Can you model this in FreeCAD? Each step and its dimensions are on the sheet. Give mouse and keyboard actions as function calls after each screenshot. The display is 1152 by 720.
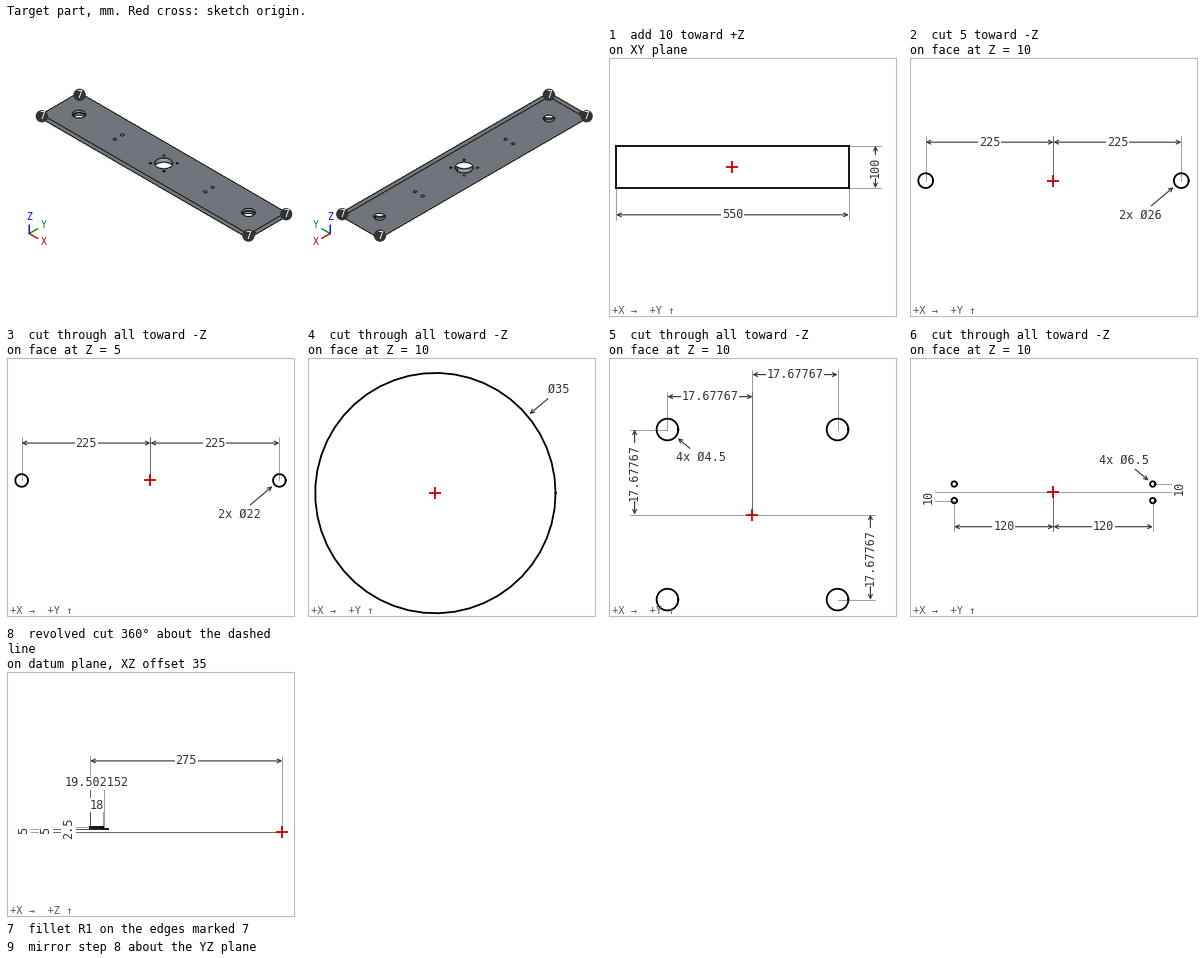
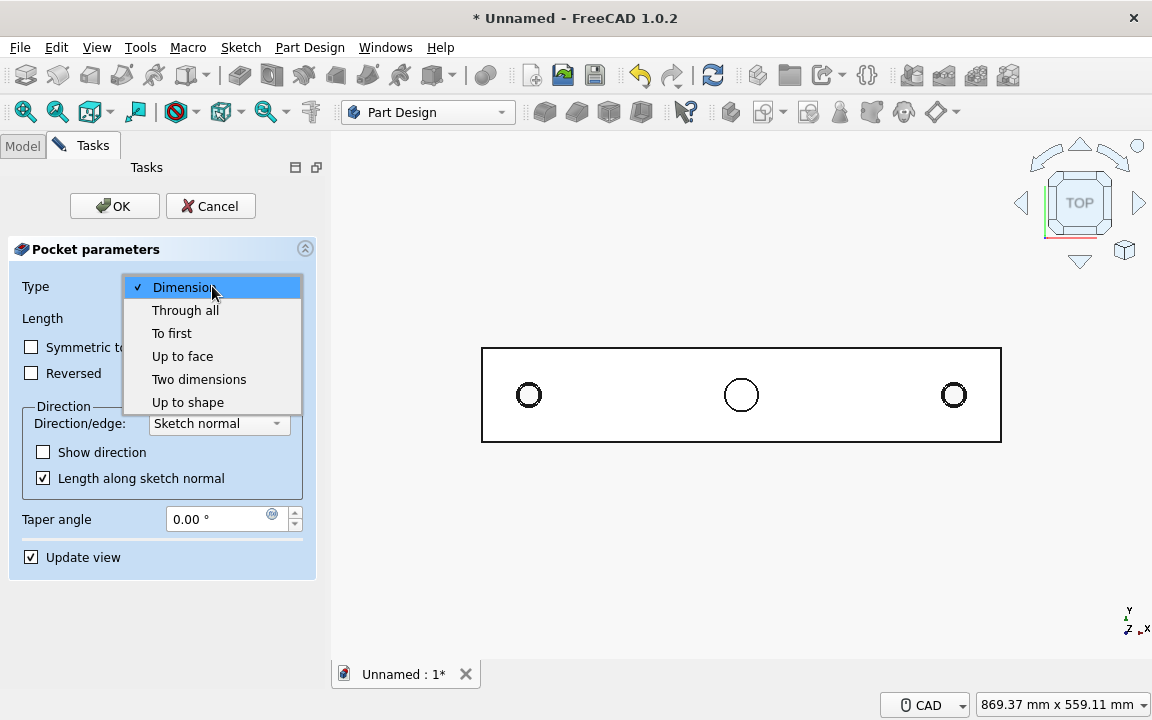
click(212, 310)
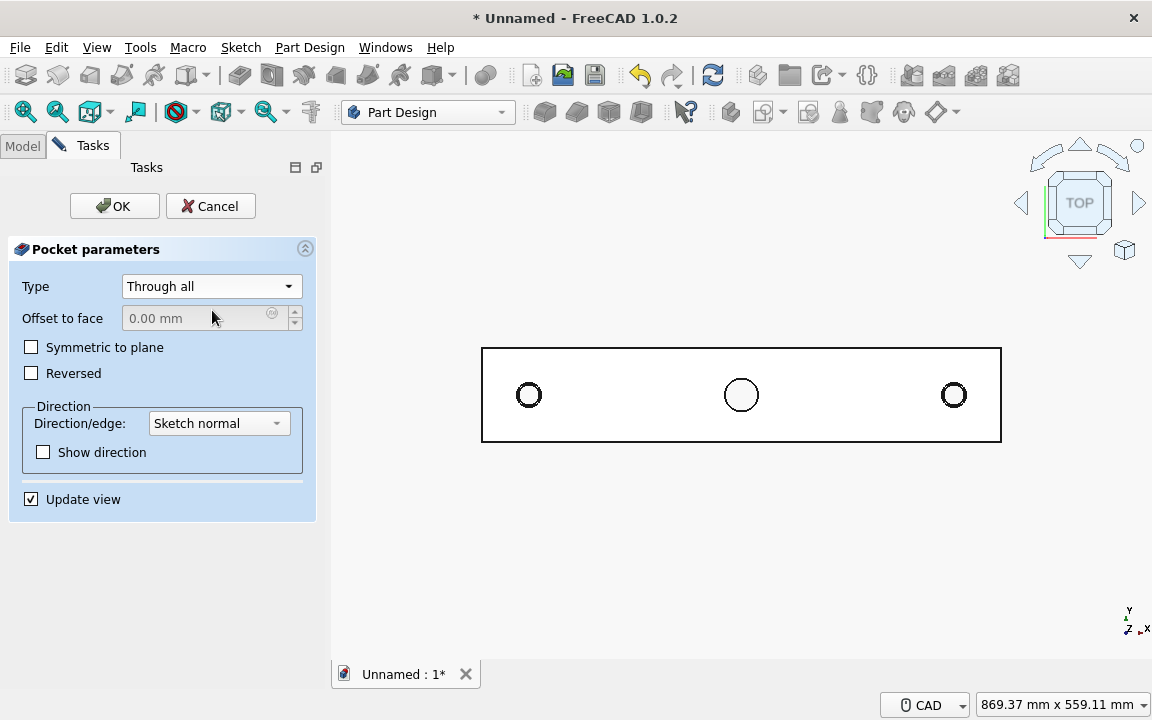
click(115, 206)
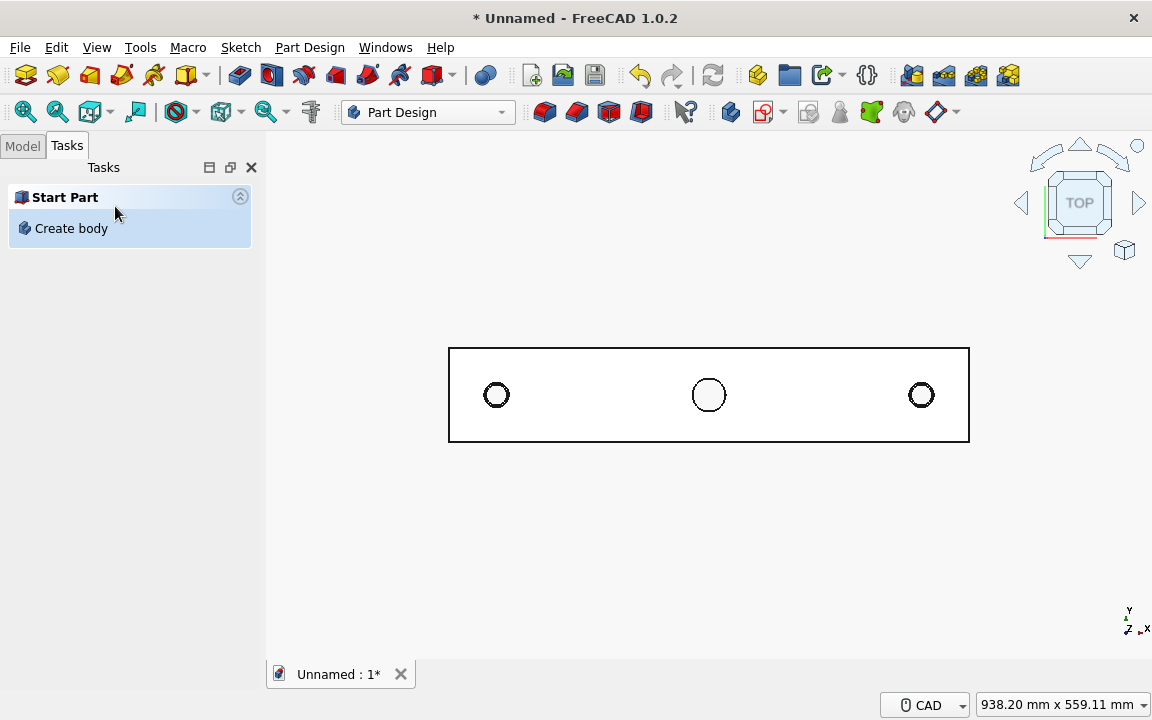
click(857, 394)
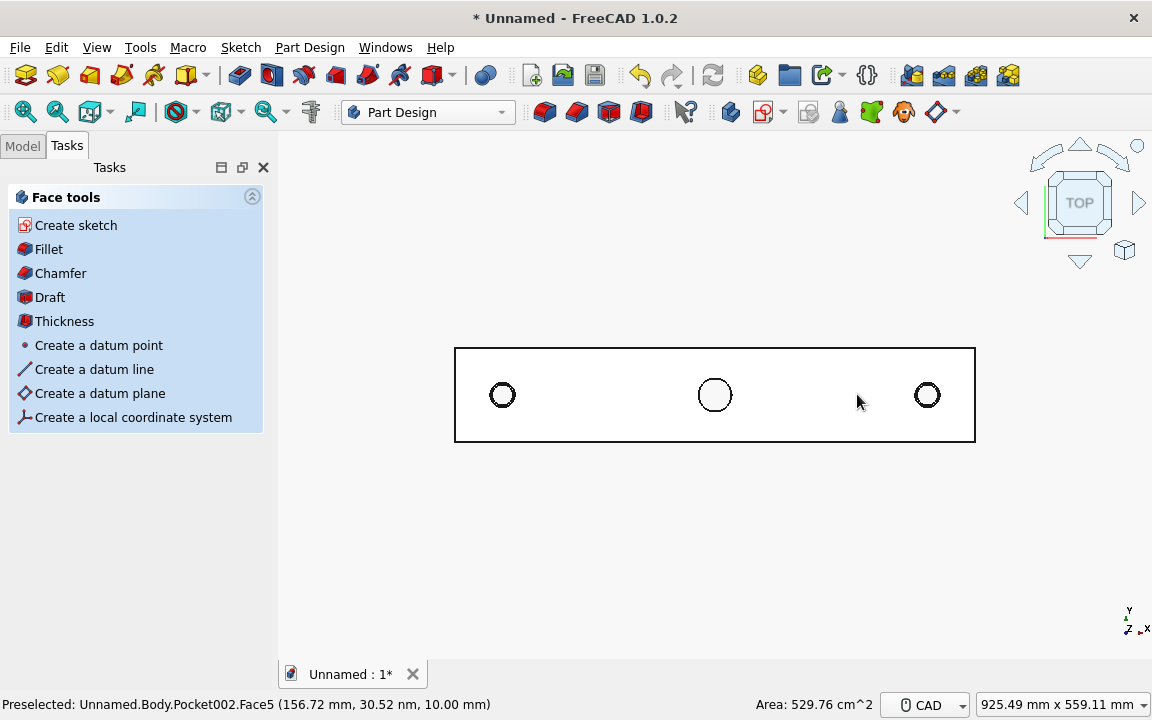
click(764, 112)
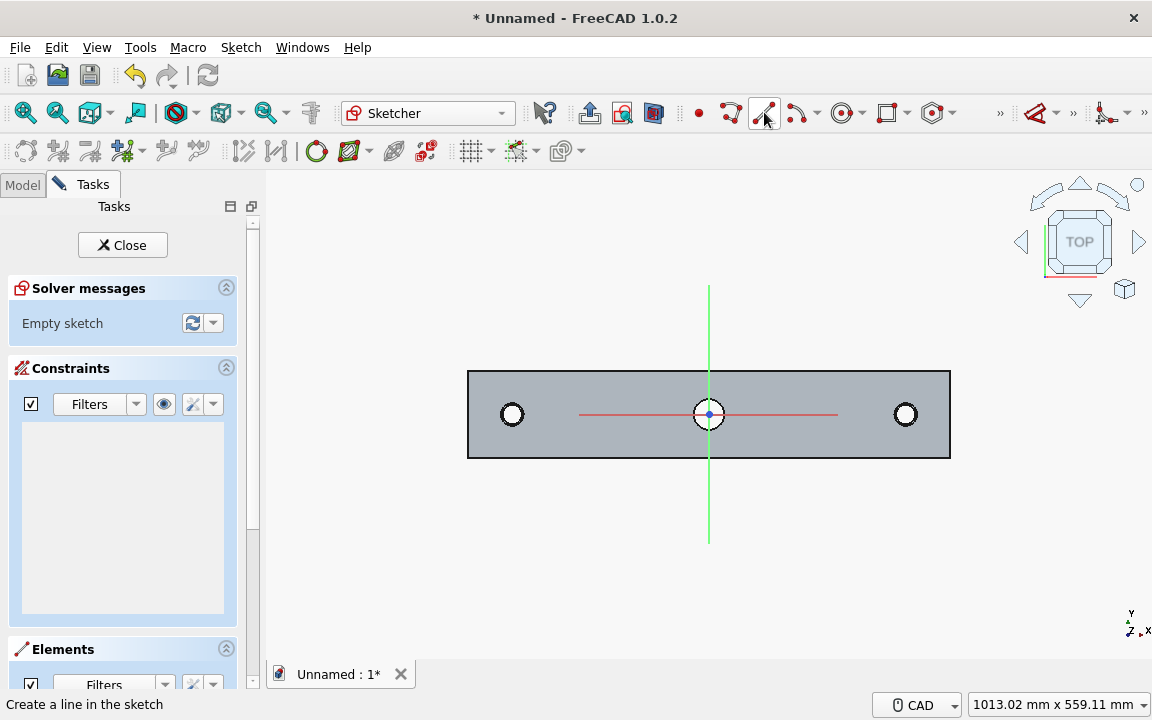
scroll(718, 415, up, 11)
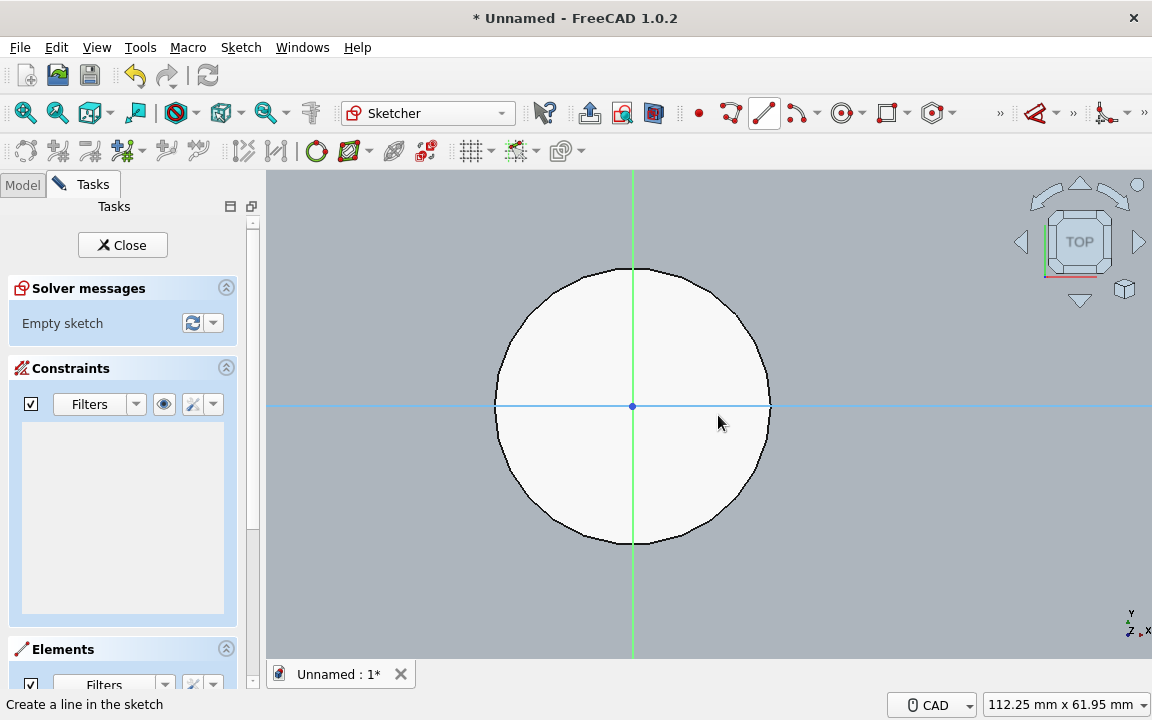
click(842, 114)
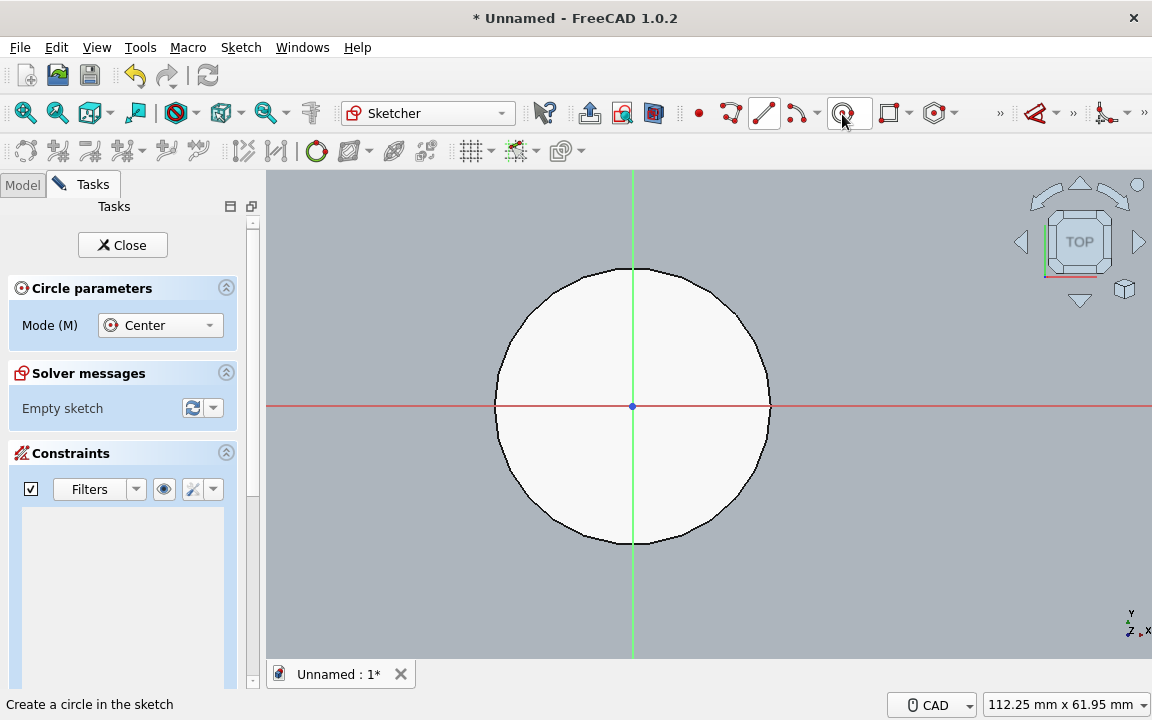
scroll(493, 267, up, 2)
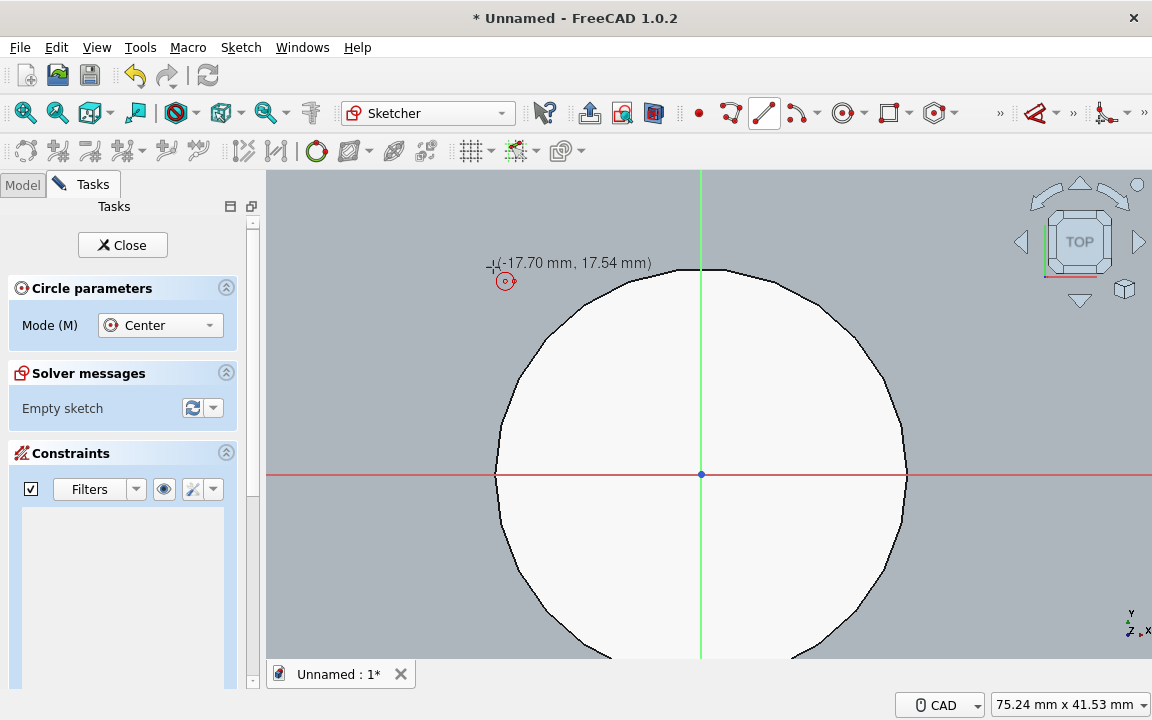
click(493, 267)
move(512, 248)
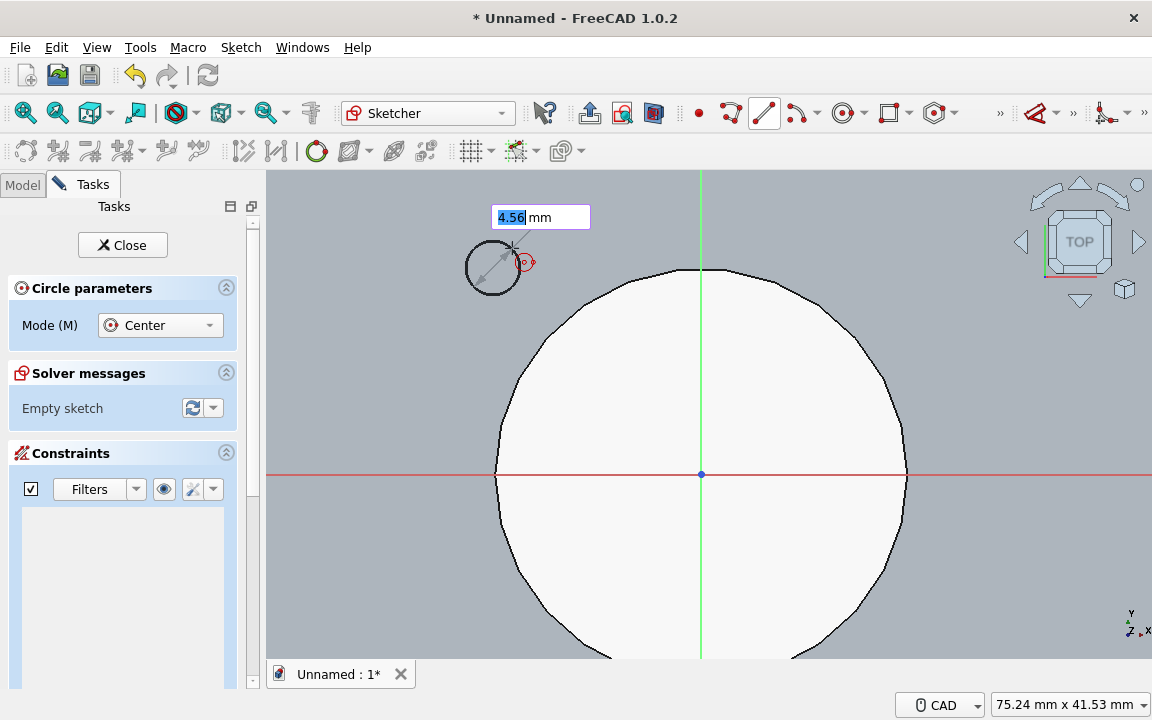
text(4.5)
key(Return)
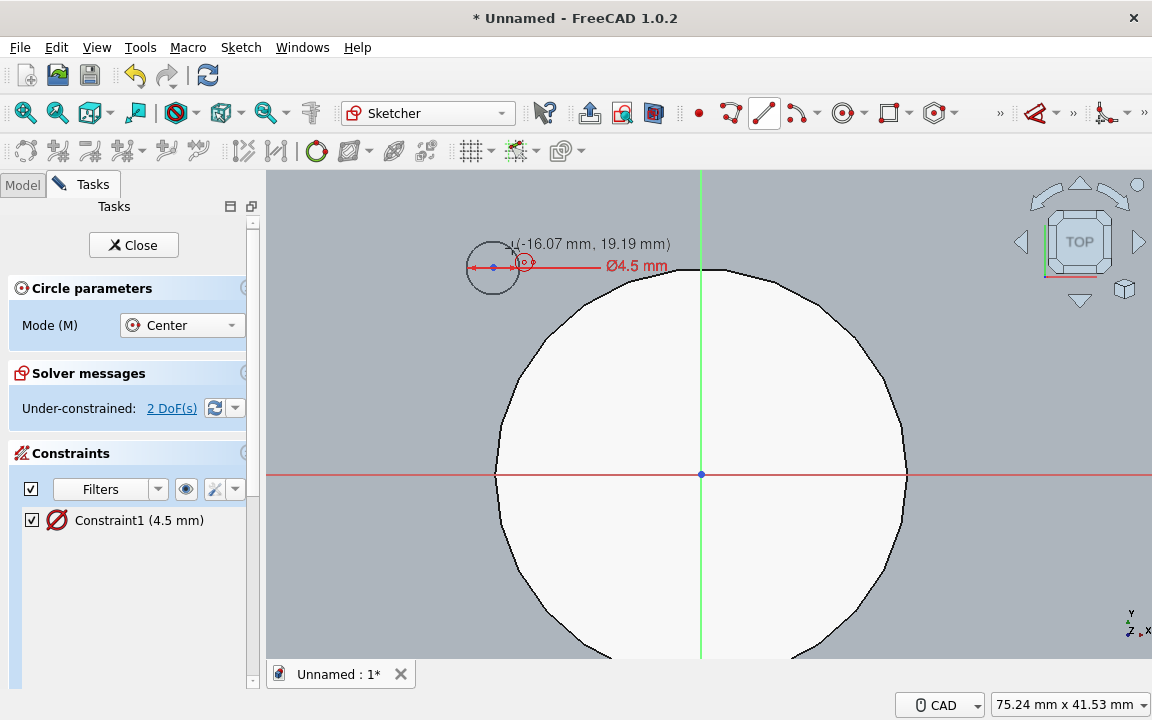
click(909, 267)
move(928, 248)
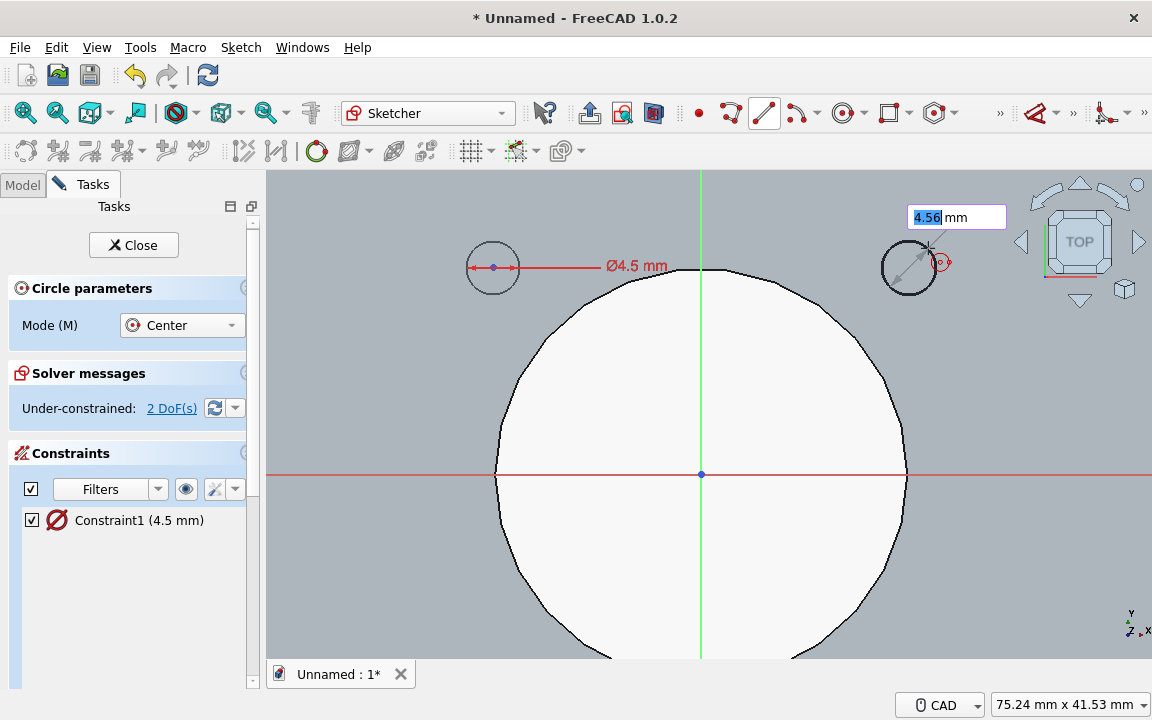
text(4.5)
key(Return)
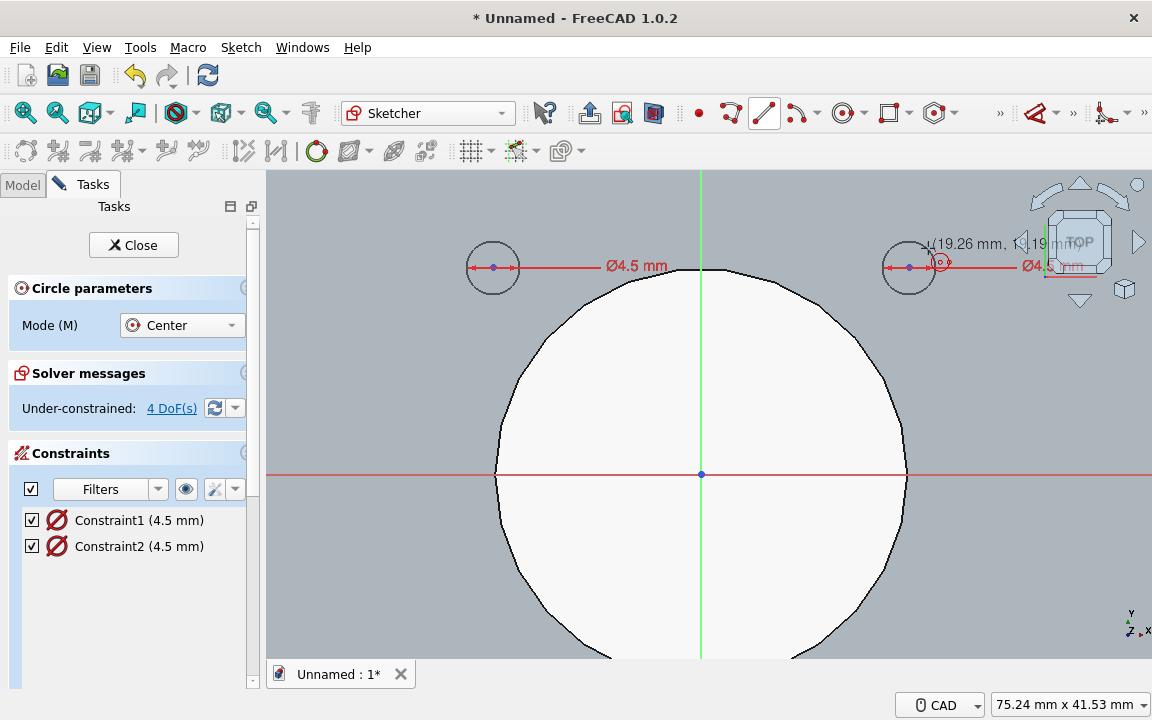
scroll(517, 292, down, 2)